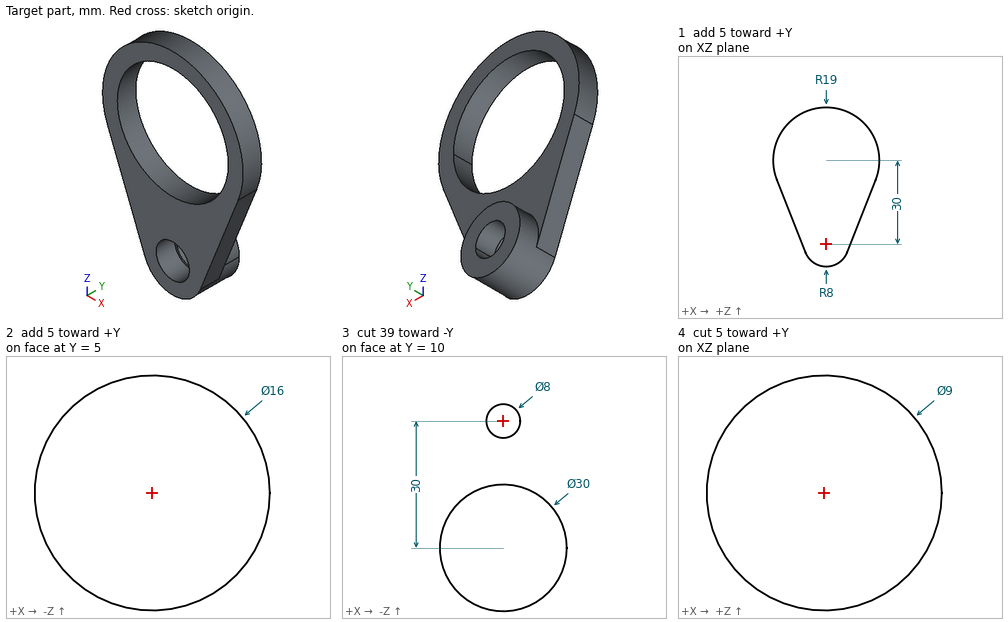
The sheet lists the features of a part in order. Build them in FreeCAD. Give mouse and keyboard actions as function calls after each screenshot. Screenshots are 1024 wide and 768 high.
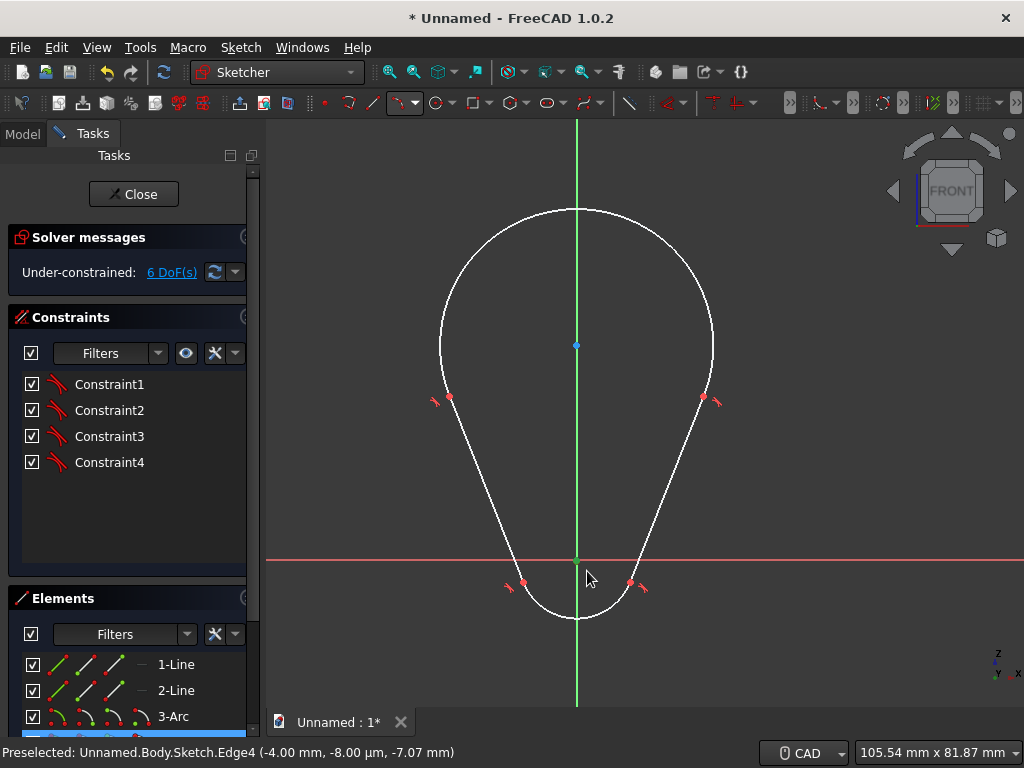
click(714, 104)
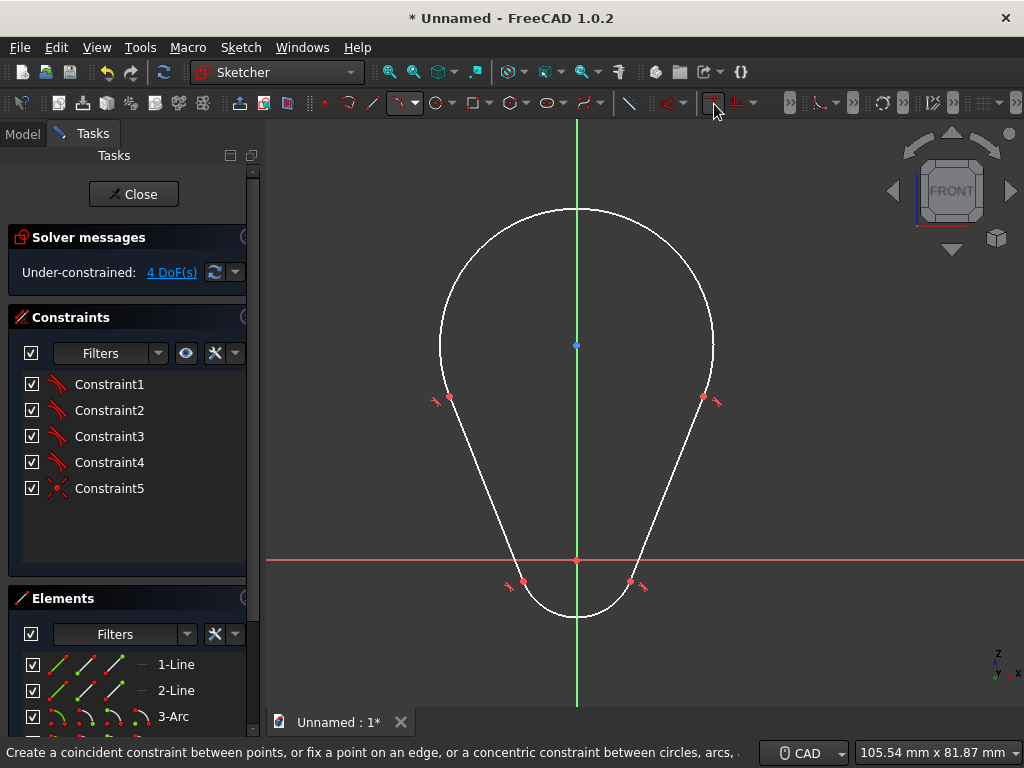
click(577, 345)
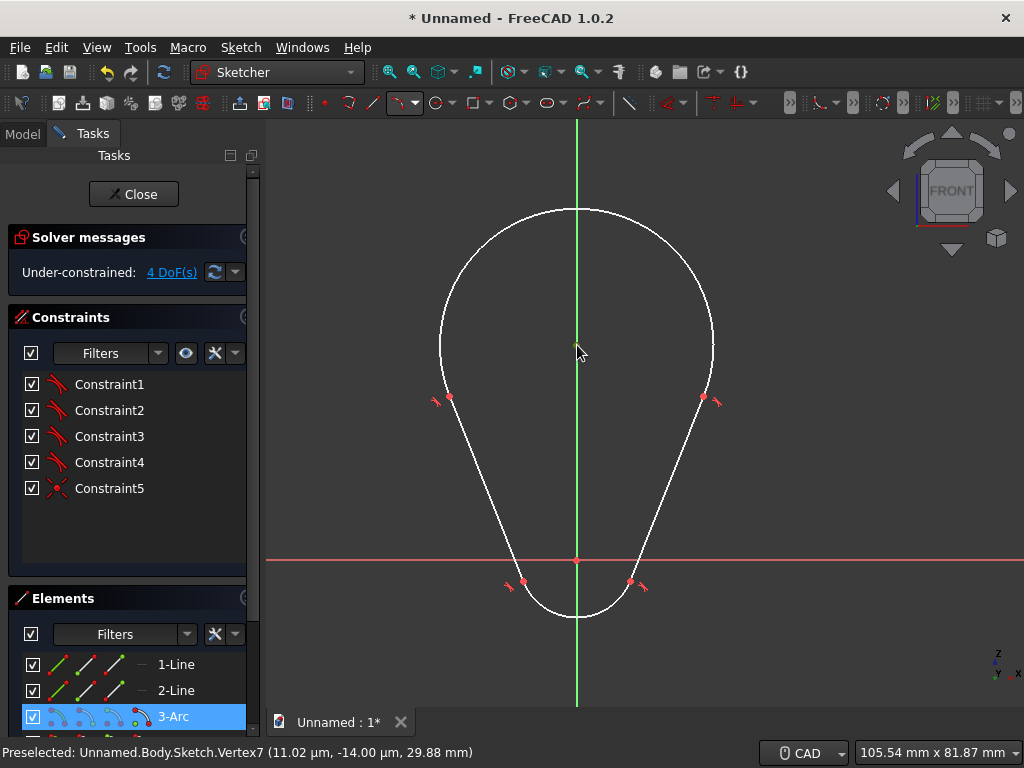
click(577, 527)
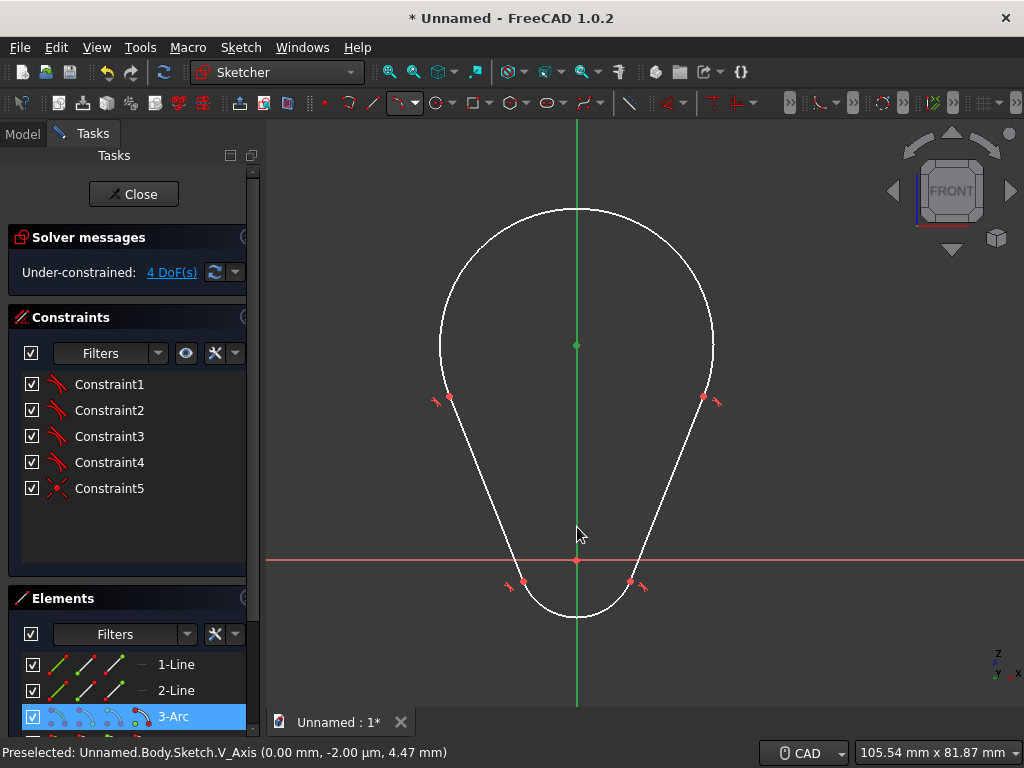
click(714, 104)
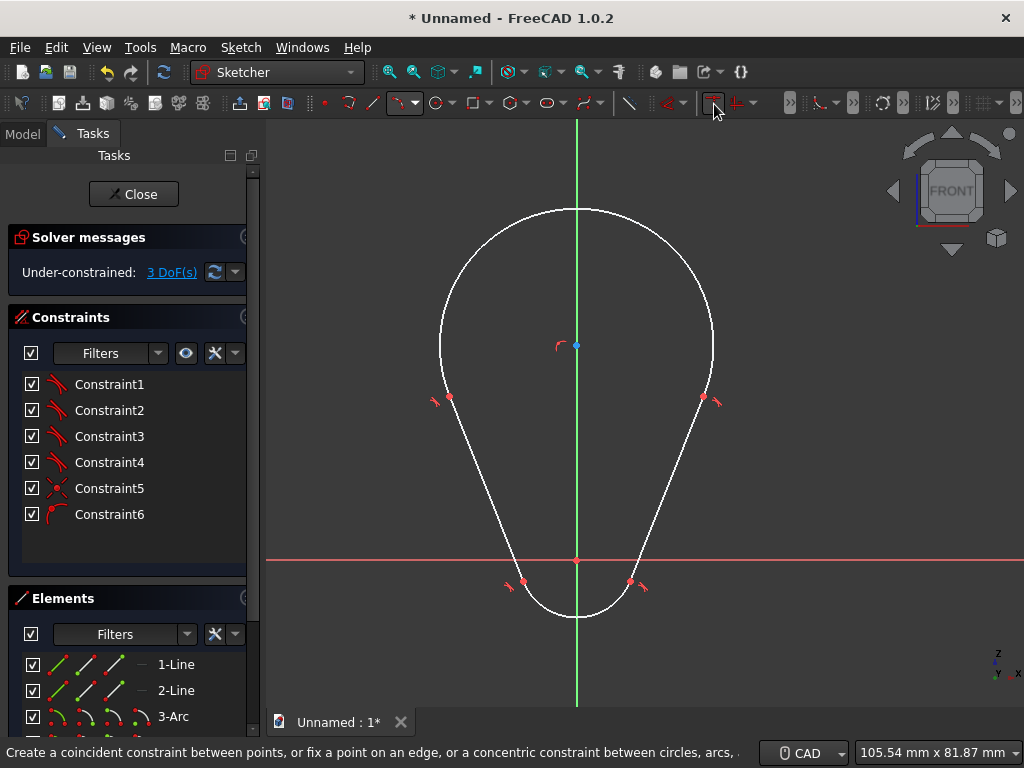
click(668, 104)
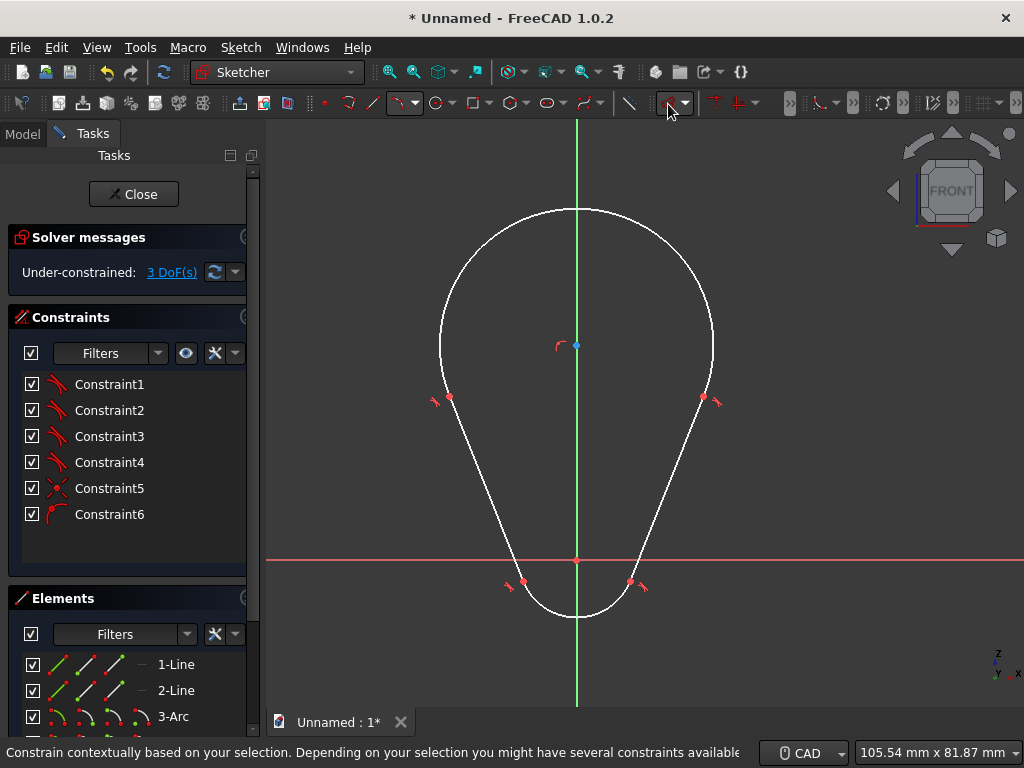
click(673, 248)
click(695, 225)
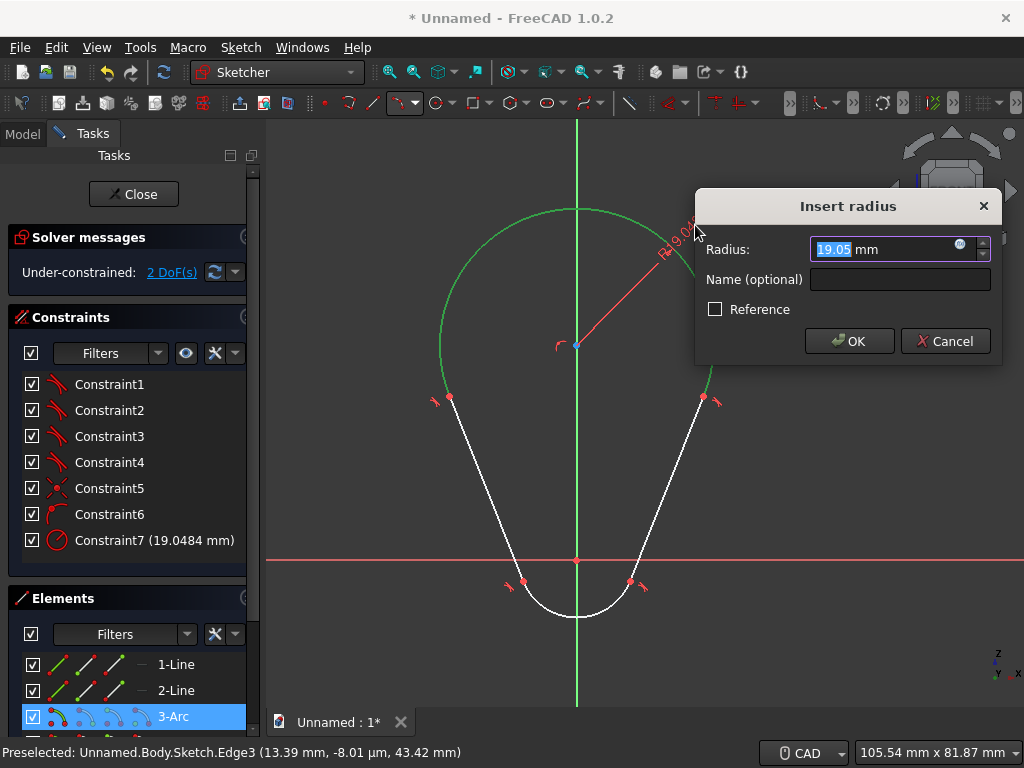
text(19)
key(Return)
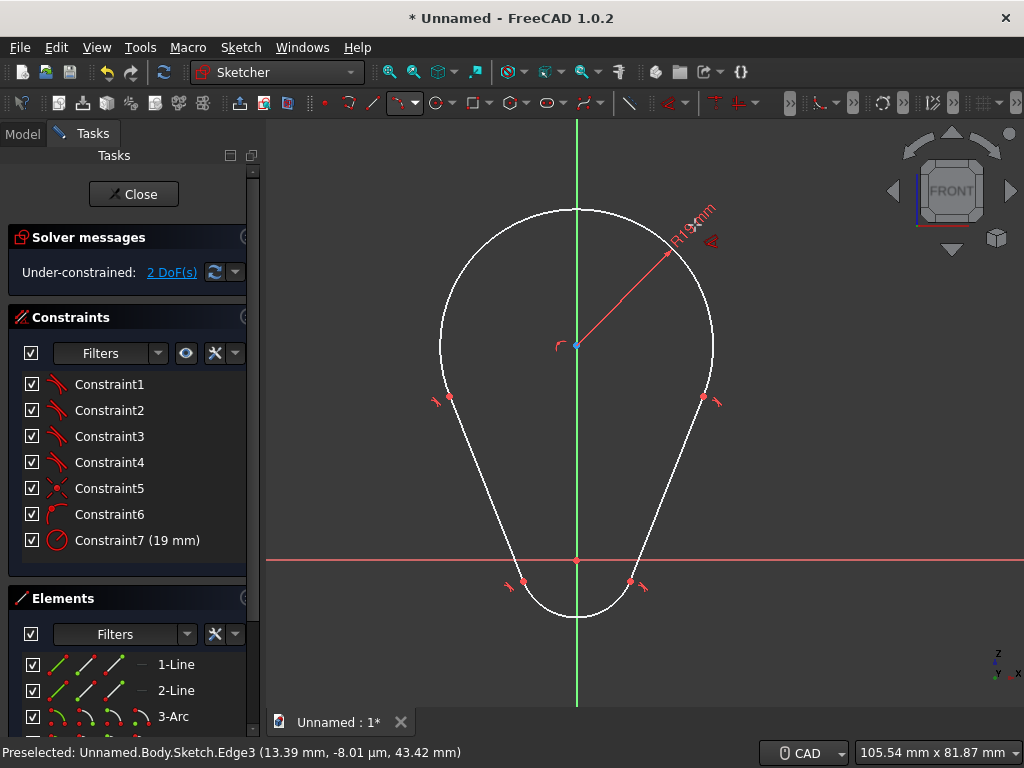
click(550, 611)
click(535, 639)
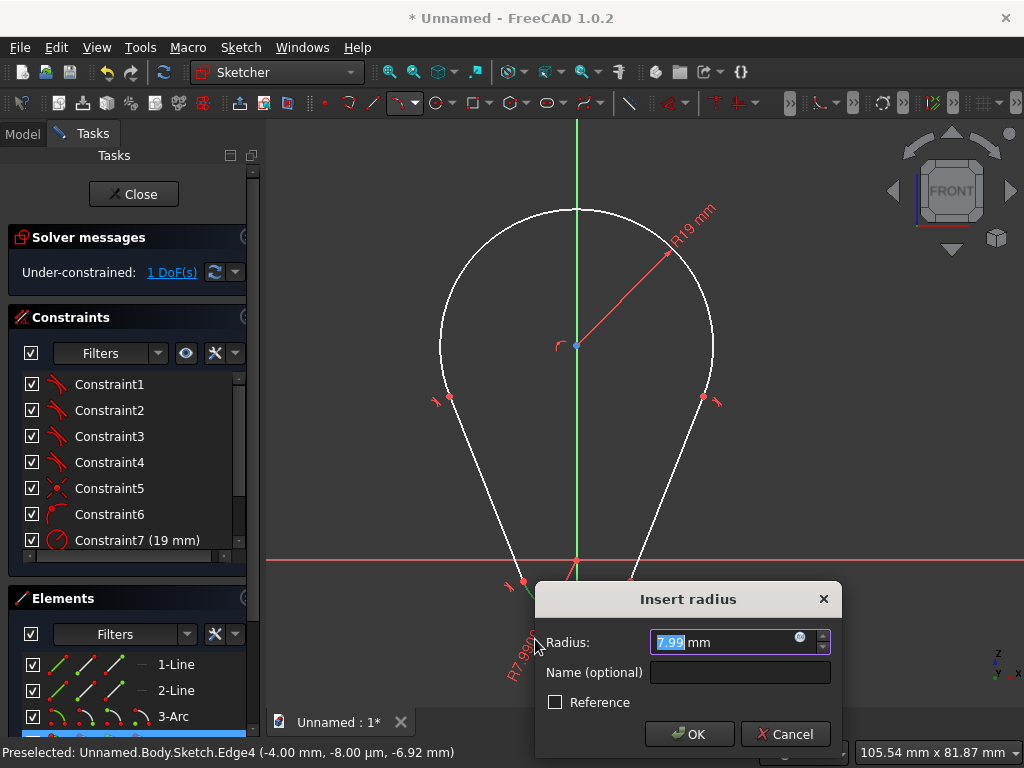
text(8)
key(Return)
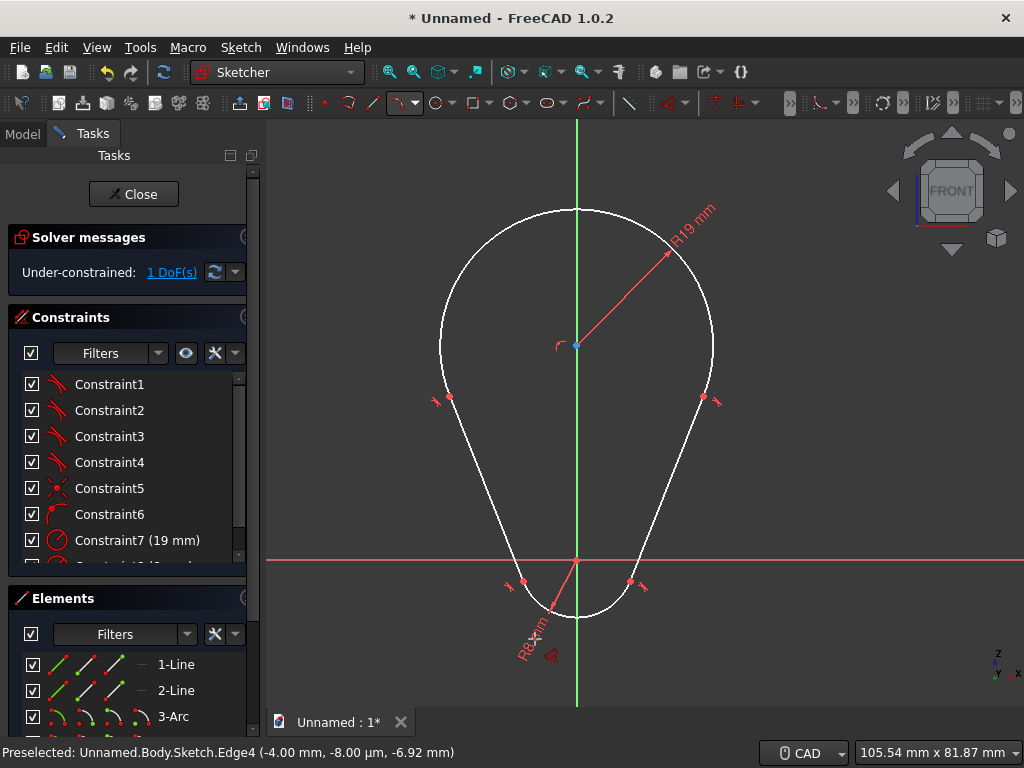
click(577, 346)
click(611, 453)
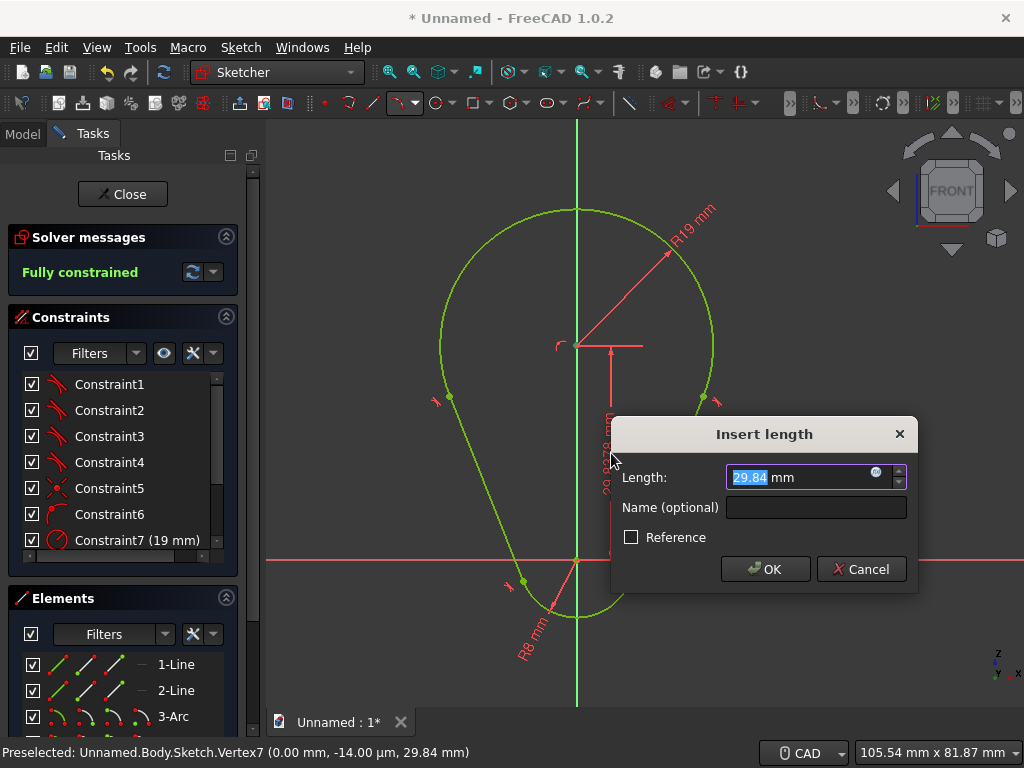
text(30)
key(Return)
key(Escape)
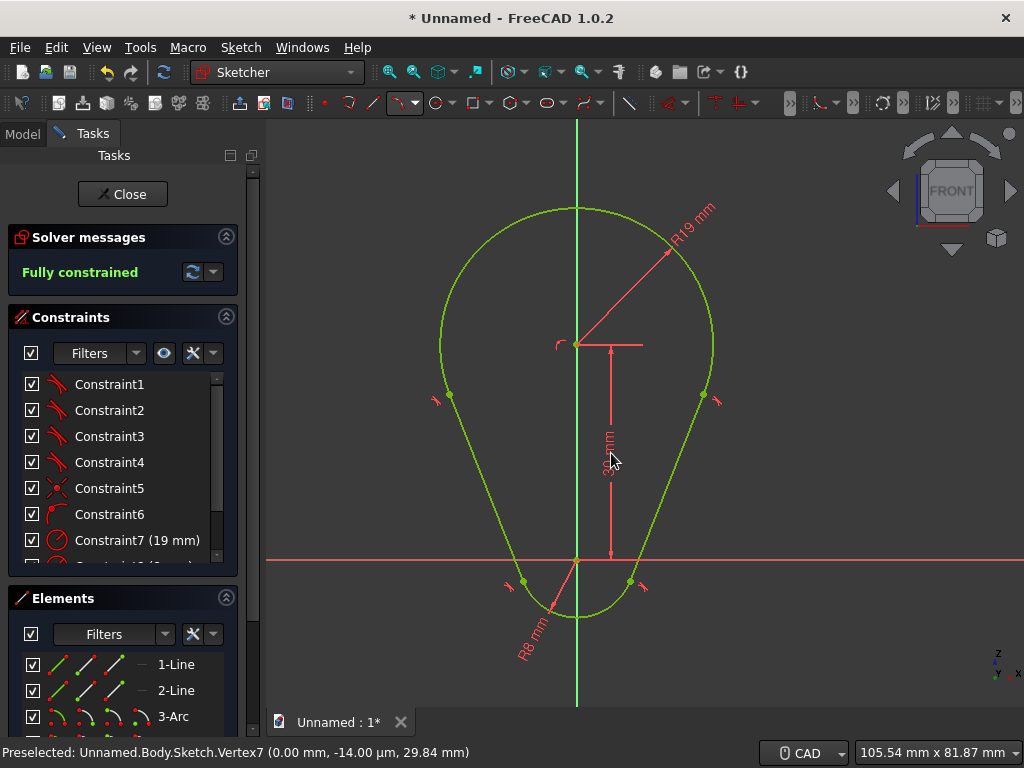
click(123, 194)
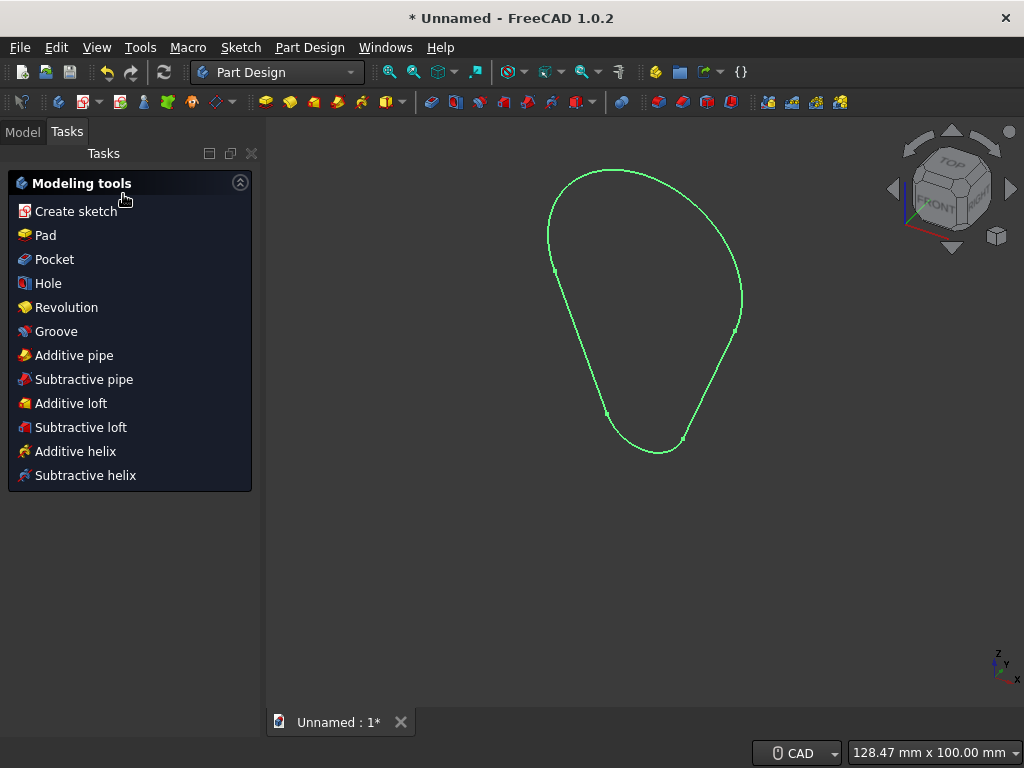
click(266, 102)